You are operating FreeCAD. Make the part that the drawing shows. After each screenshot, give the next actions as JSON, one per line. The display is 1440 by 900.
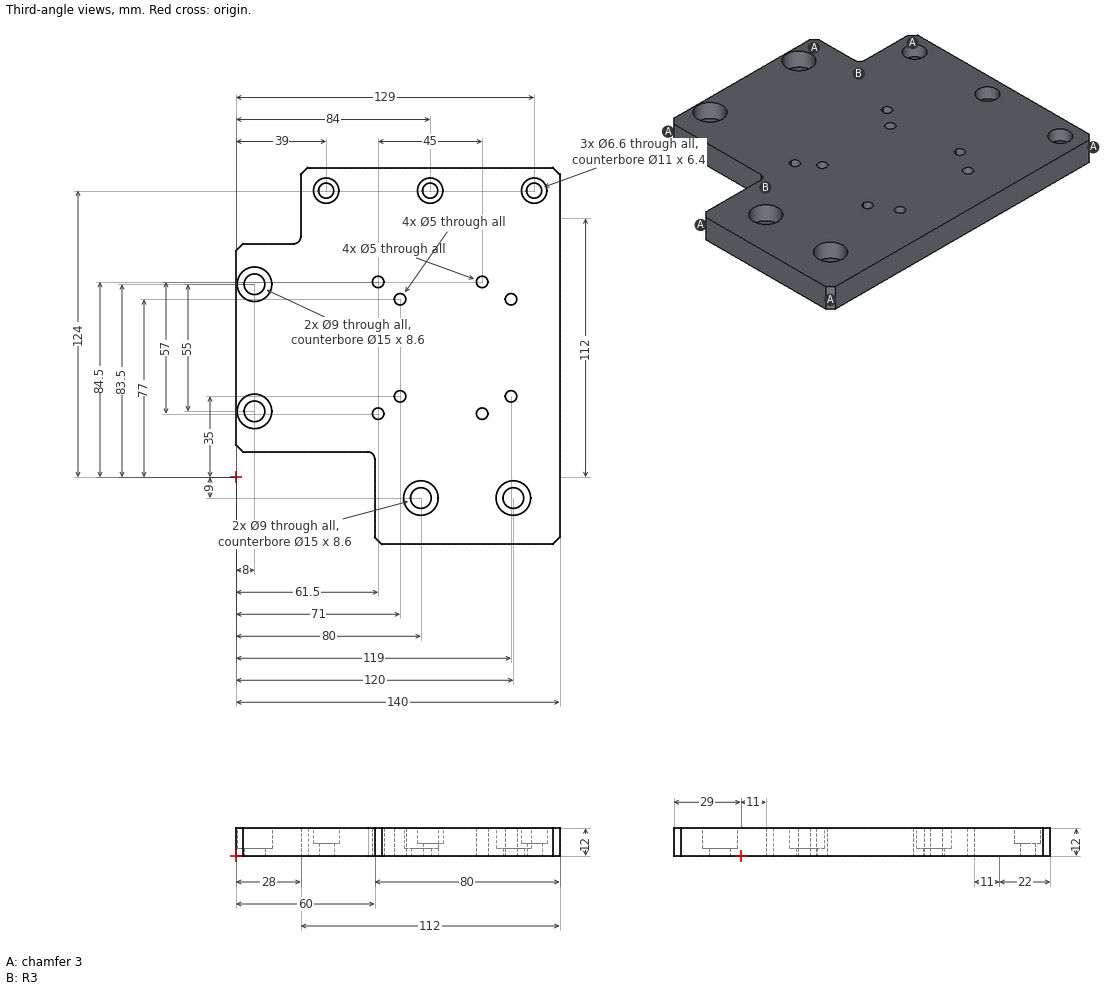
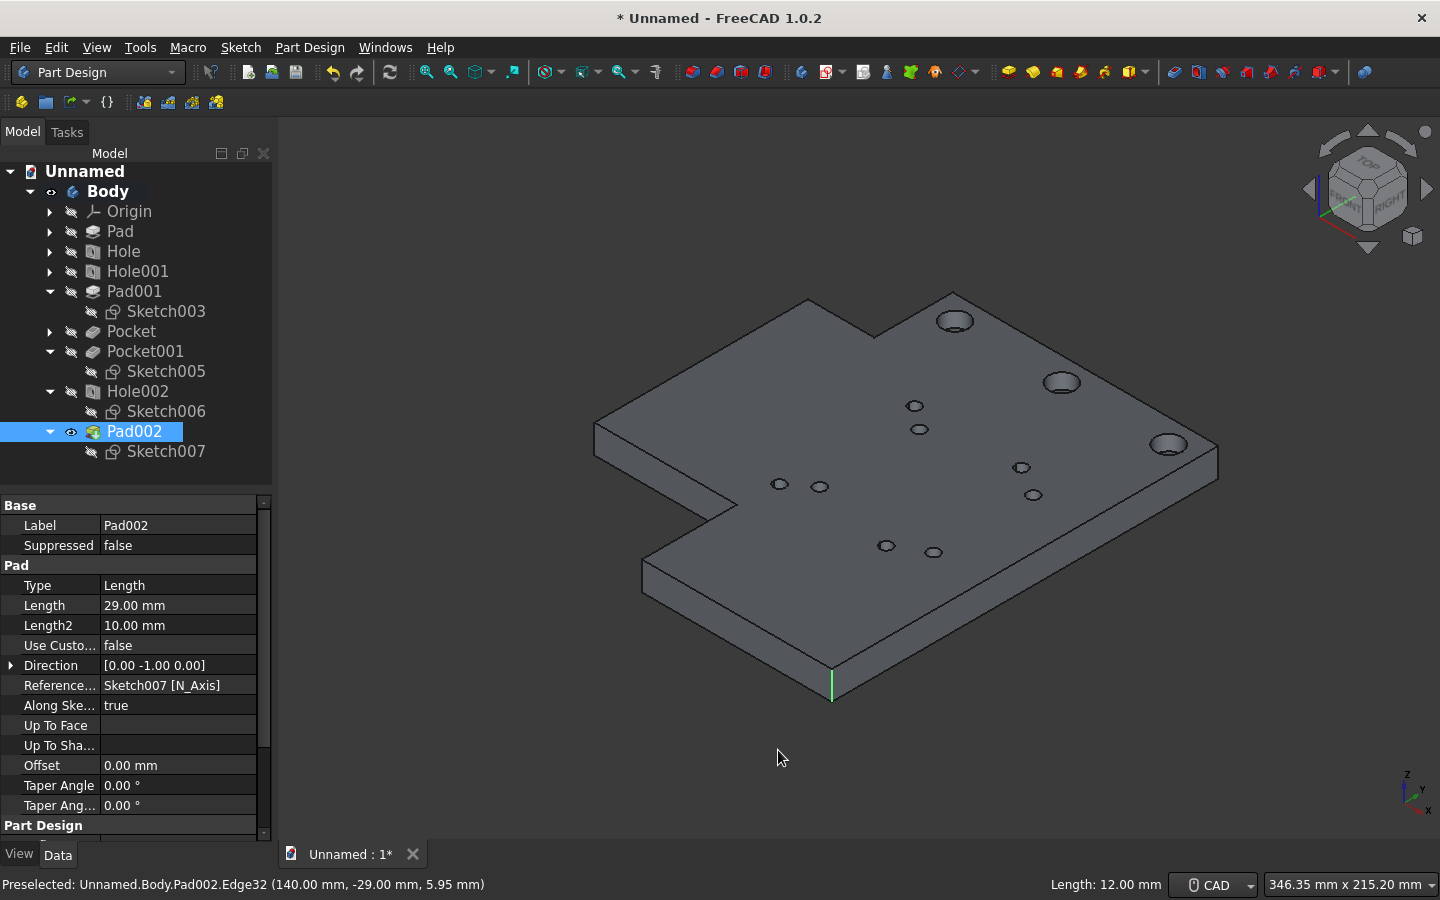
{"action": "key", "text": "1"}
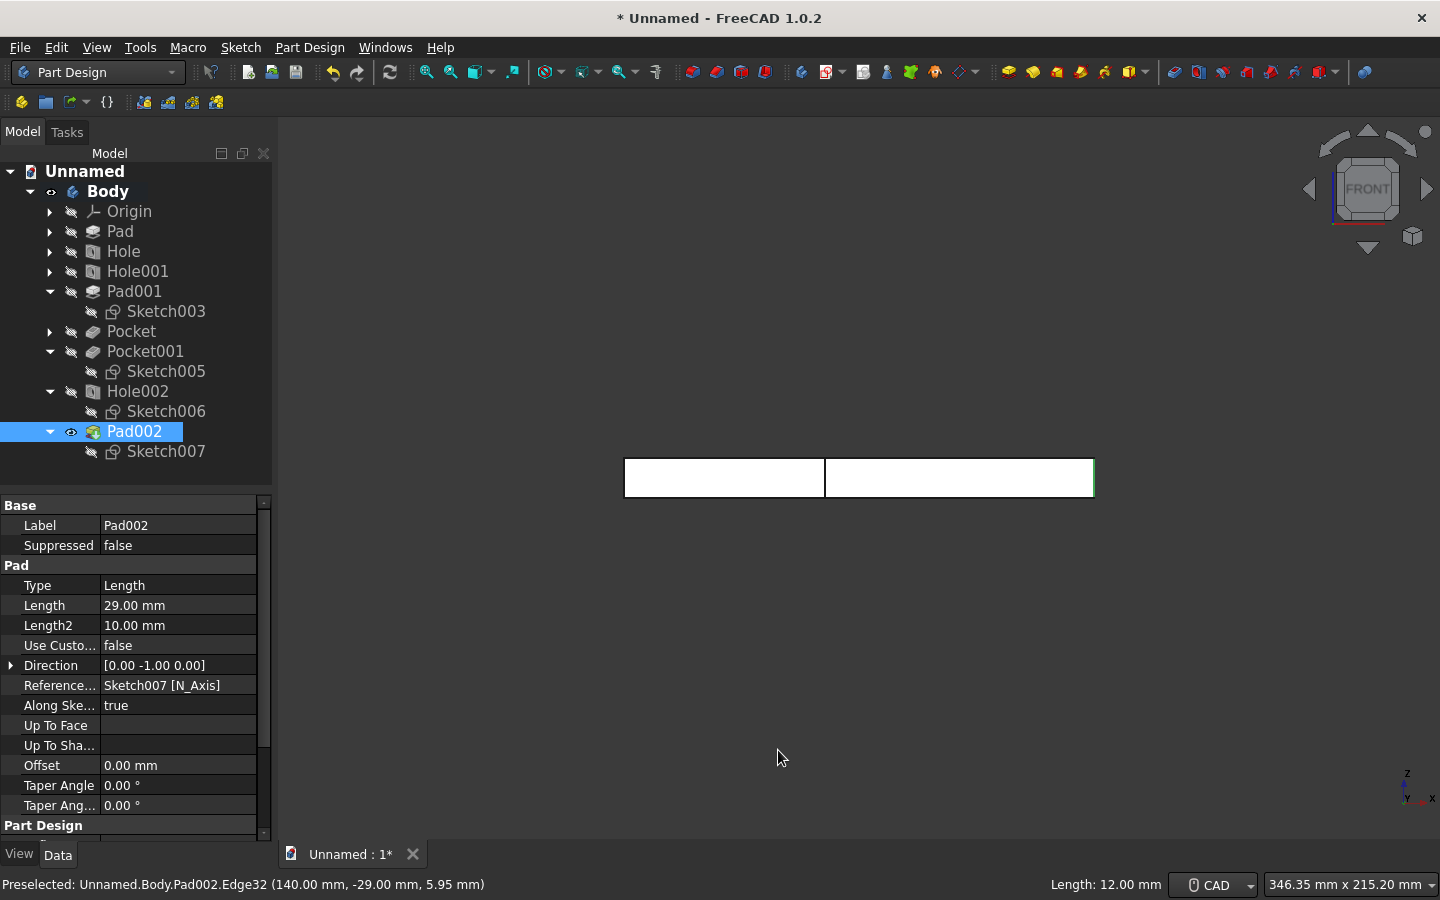
{"action": "left_click", "coordinate": [428, 72]}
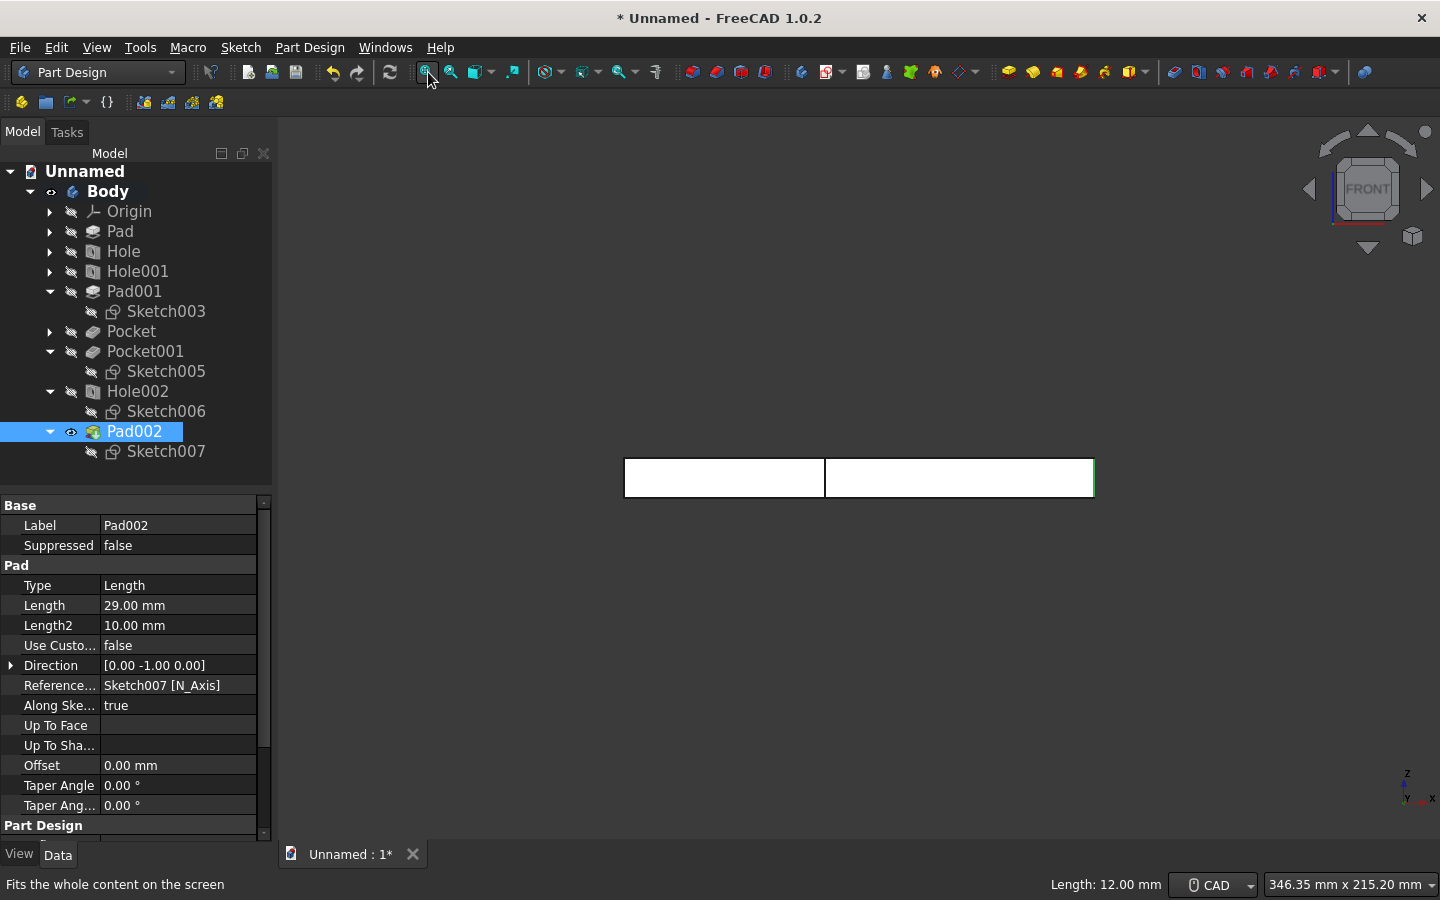
{"action": "left_click", "coordinate": [825, 477], "text": "ctrl"}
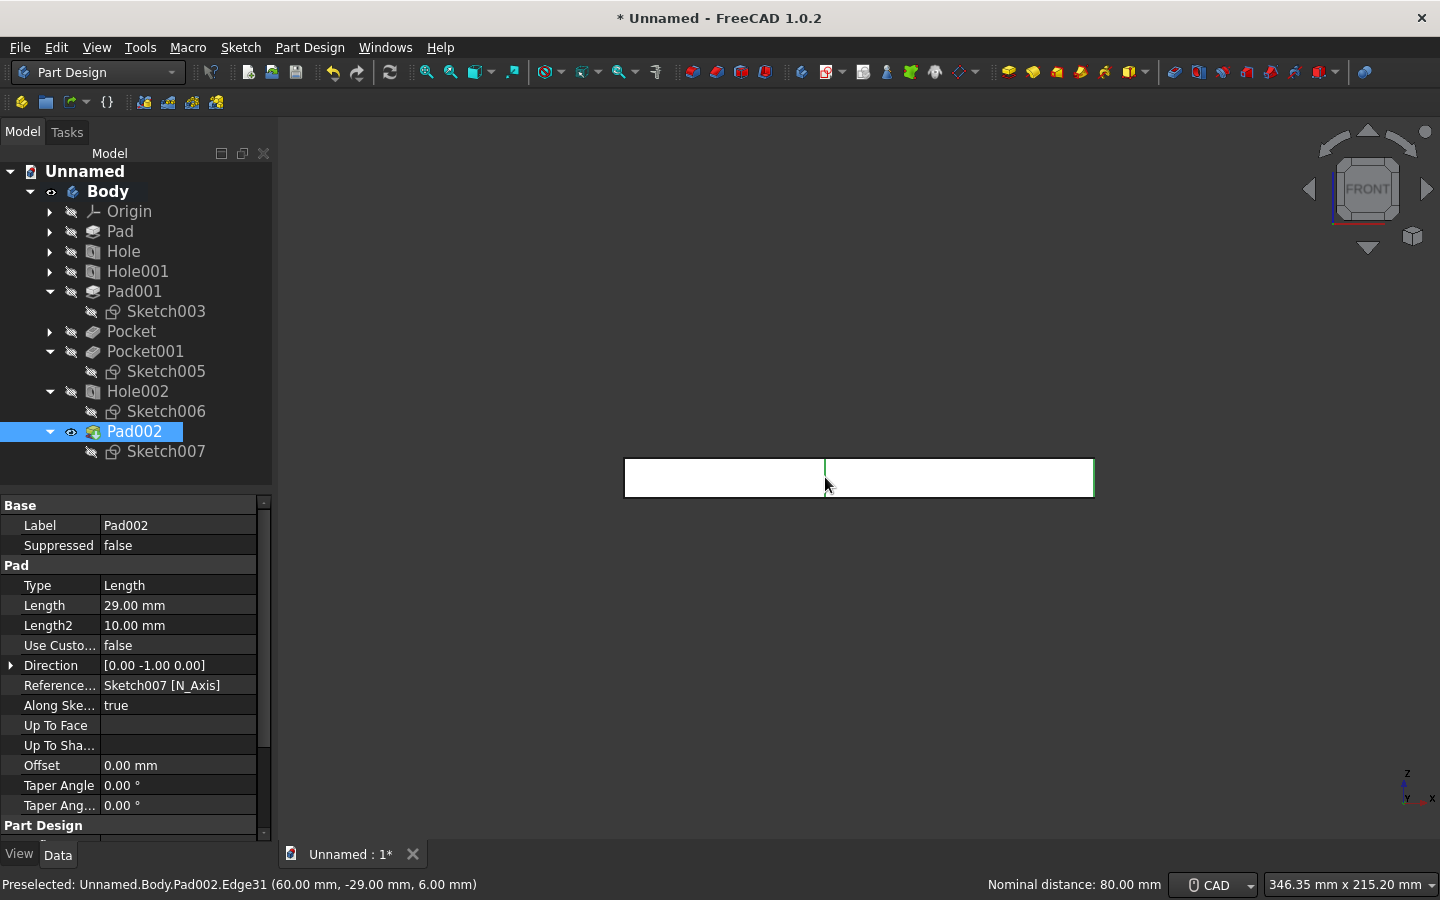
{"action": "left_click", "coordinate": [624, 477], "text": "ctrl"}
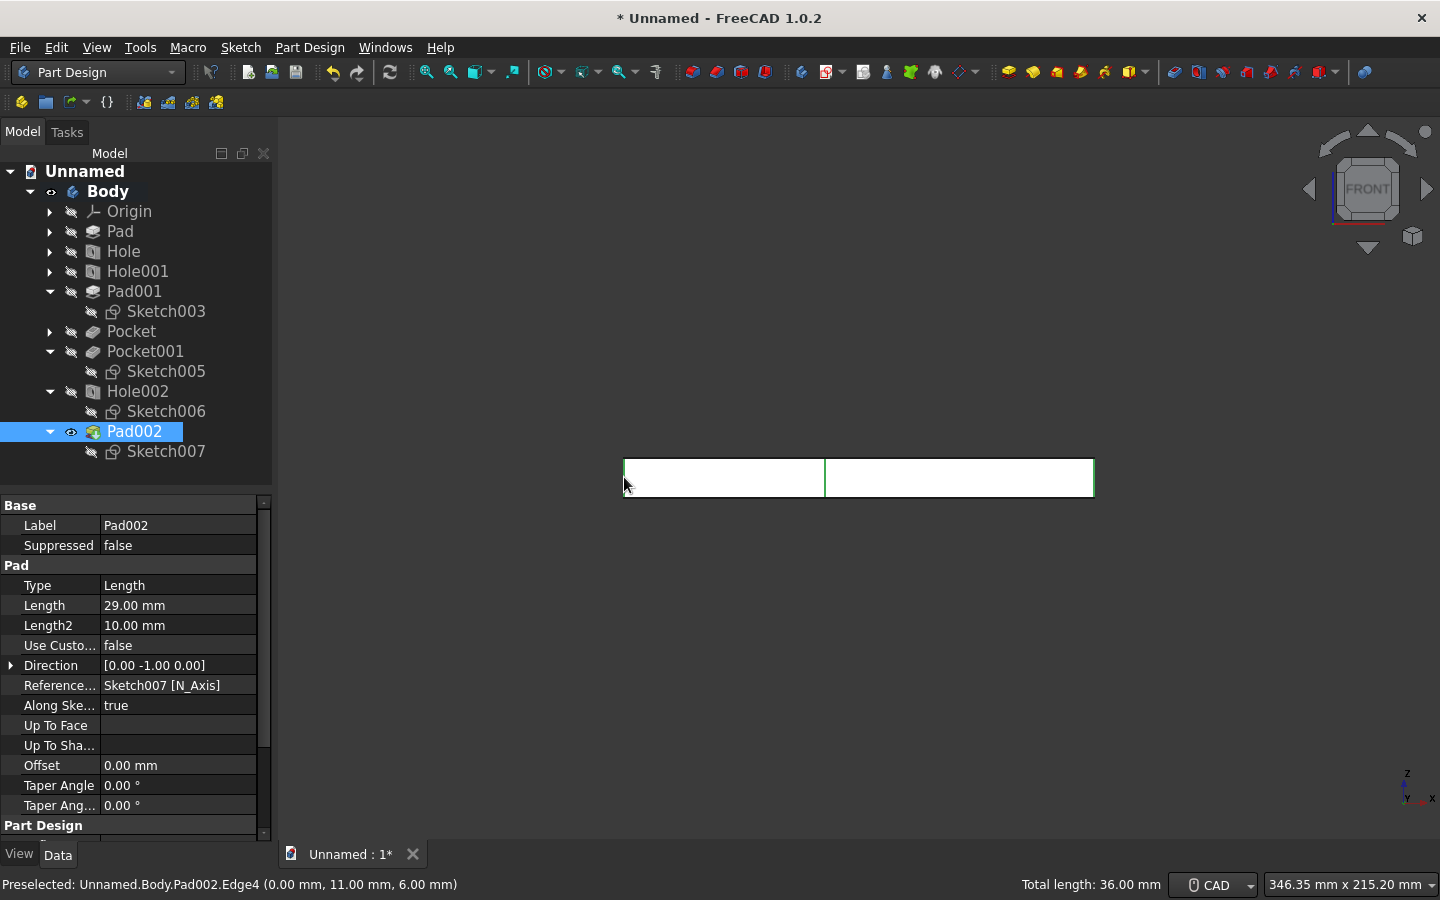
{"action": "key", "text": "3"}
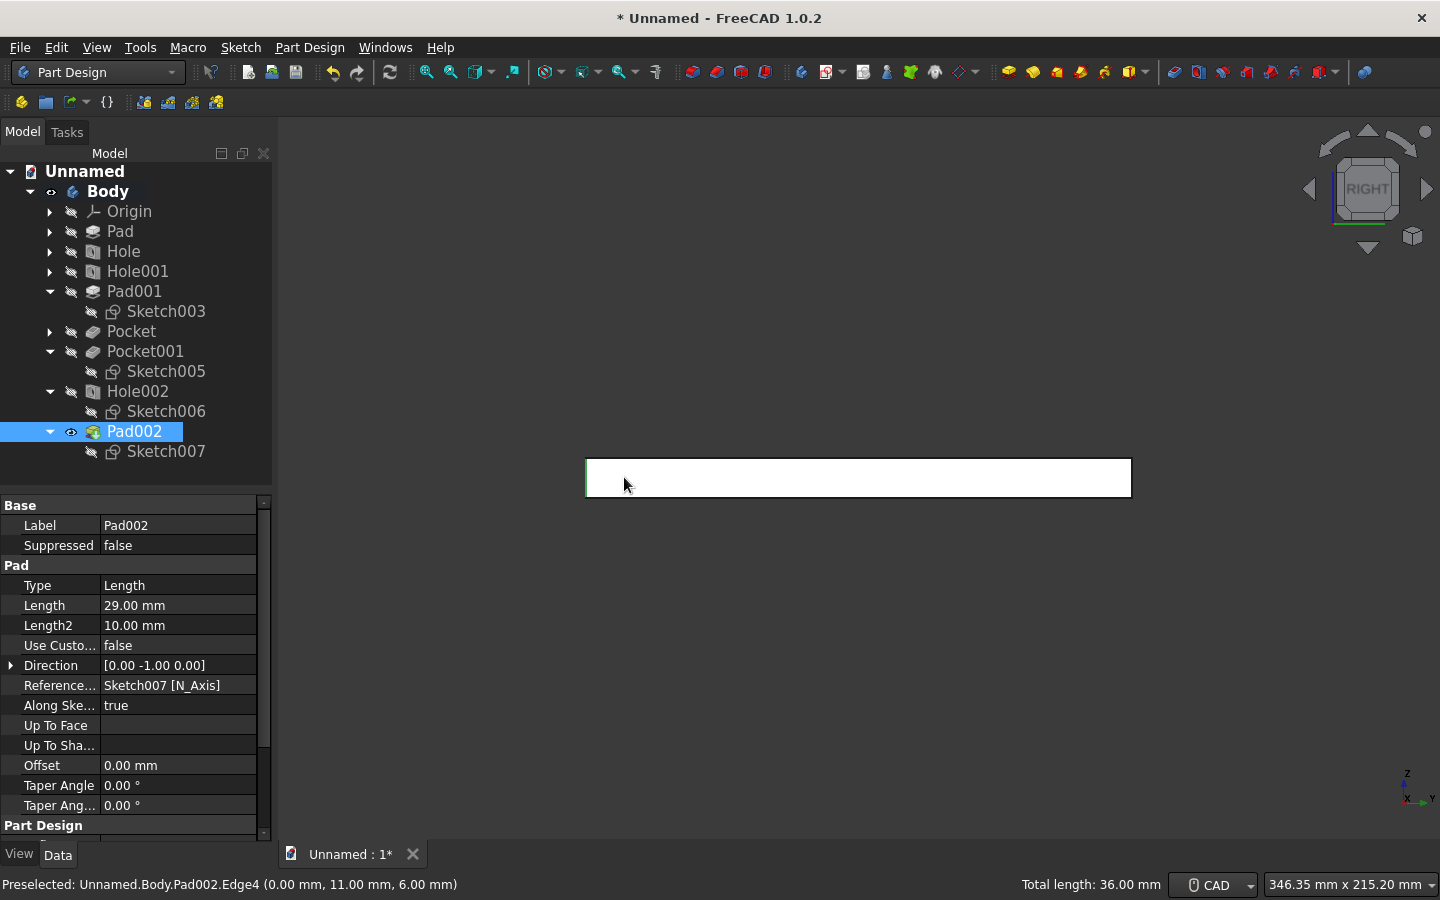
{"action": "left_click", "coordinate": [1132, 477], "text": "ctrl"}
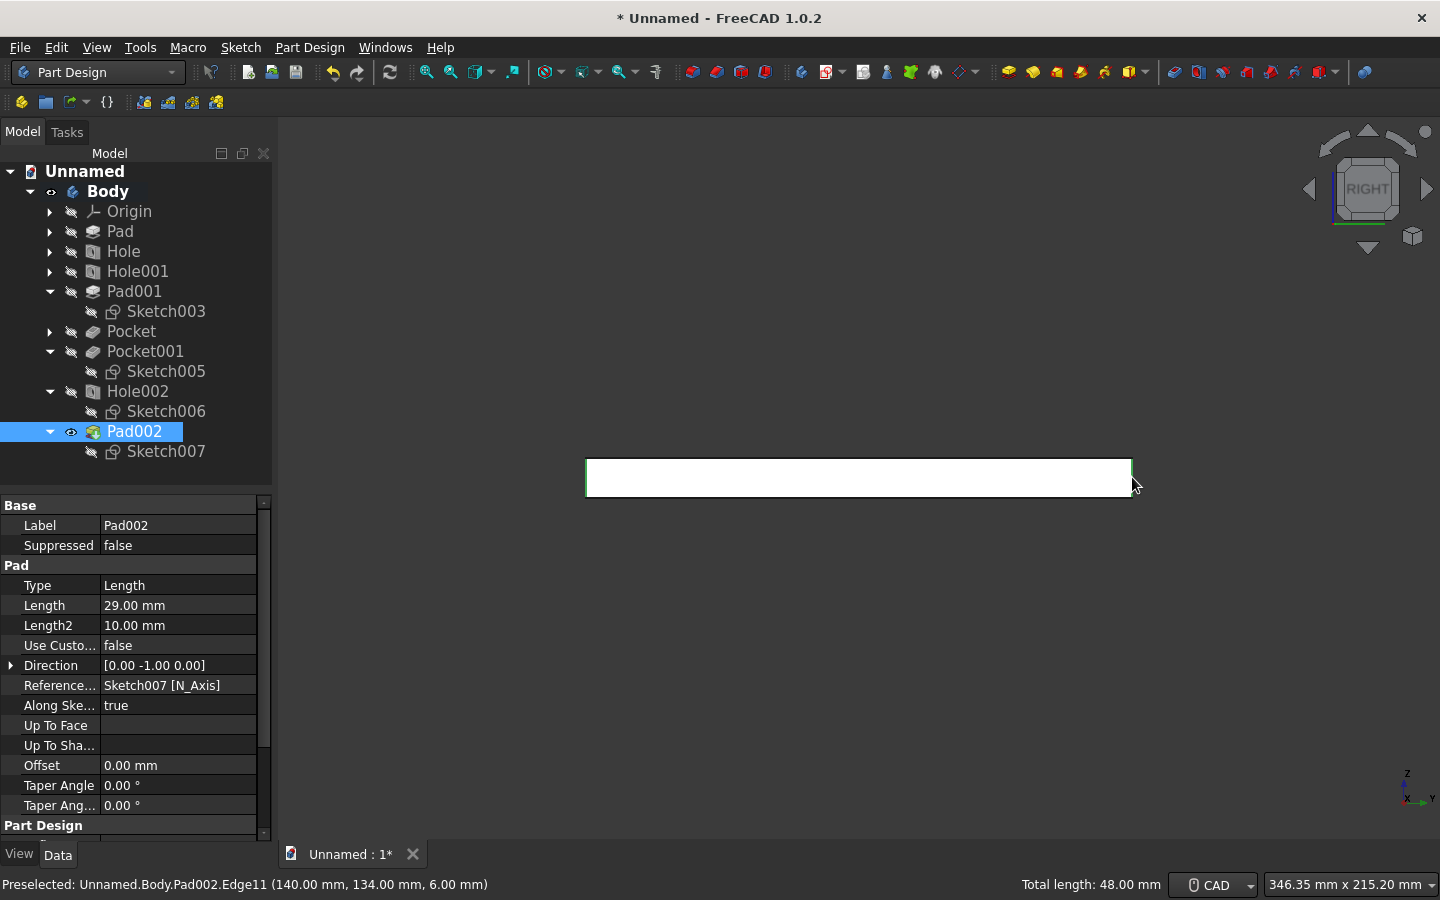
{"action": "key", "text": "5"}